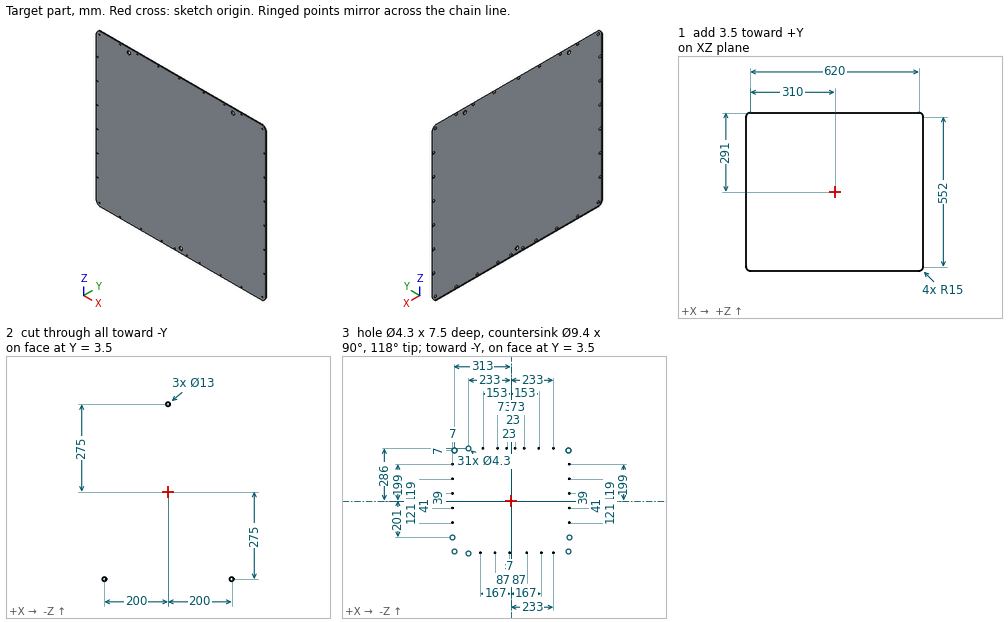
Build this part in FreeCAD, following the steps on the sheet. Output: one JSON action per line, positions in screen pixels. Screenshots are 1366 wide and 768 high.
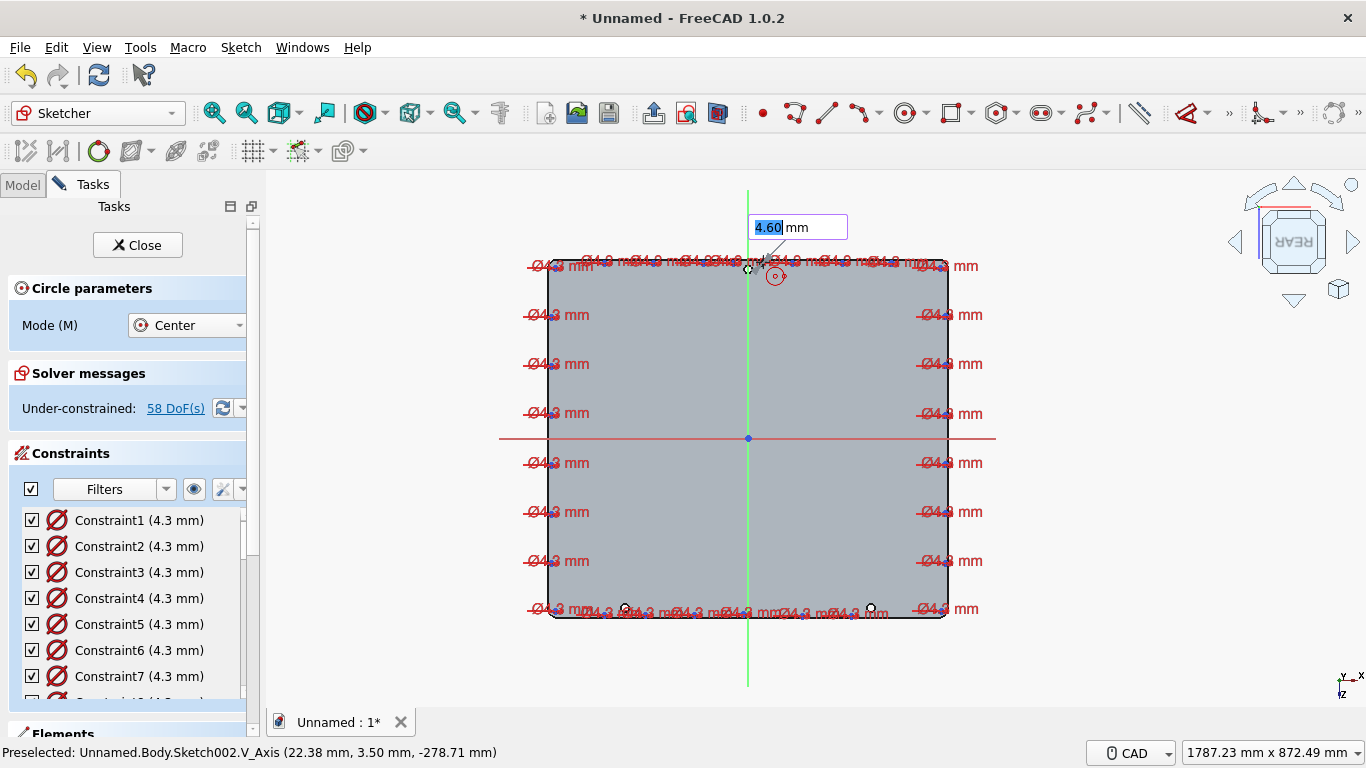
{"action": "type", "text": "4.3"}
{"action": "key", "text": "Return"}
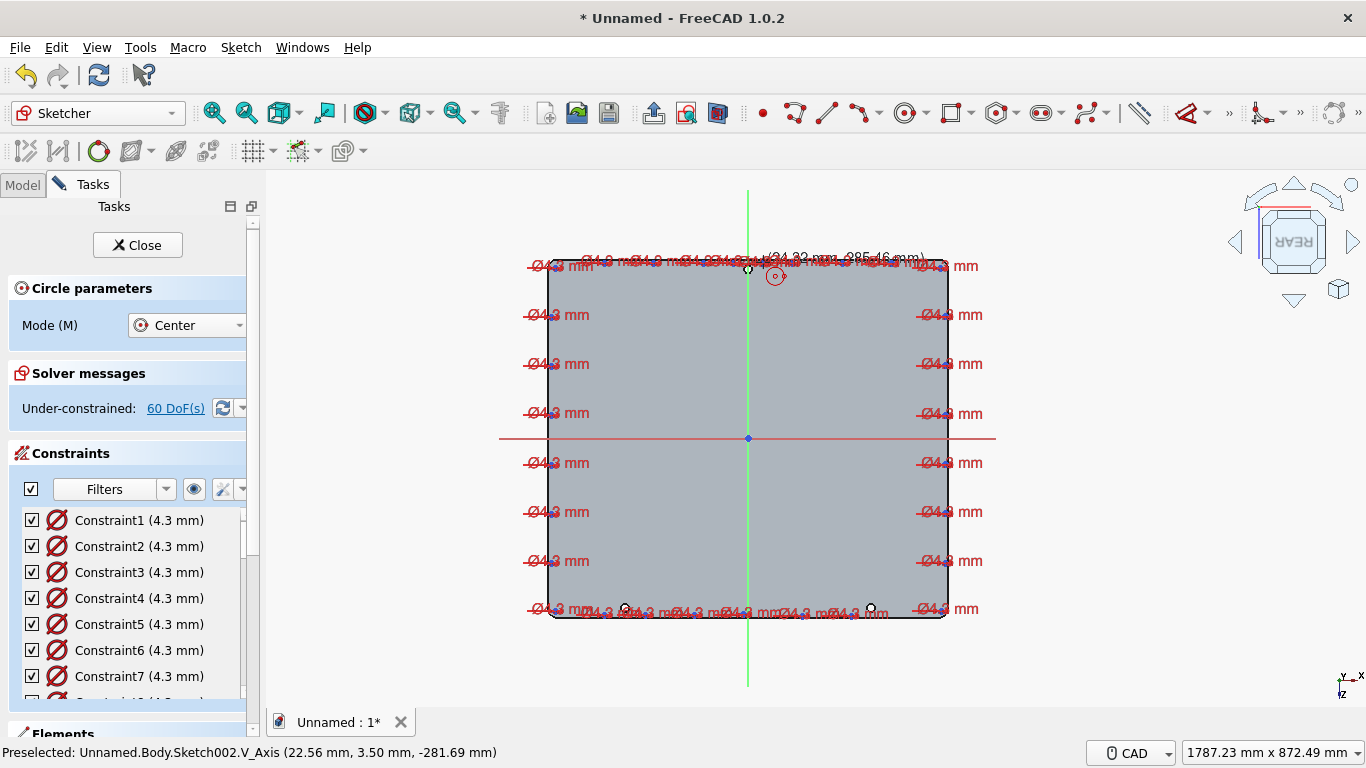
{"action": "scroll", "coordinate": [891, 615], "scroll_direction": "up", "scroll_amount": 15}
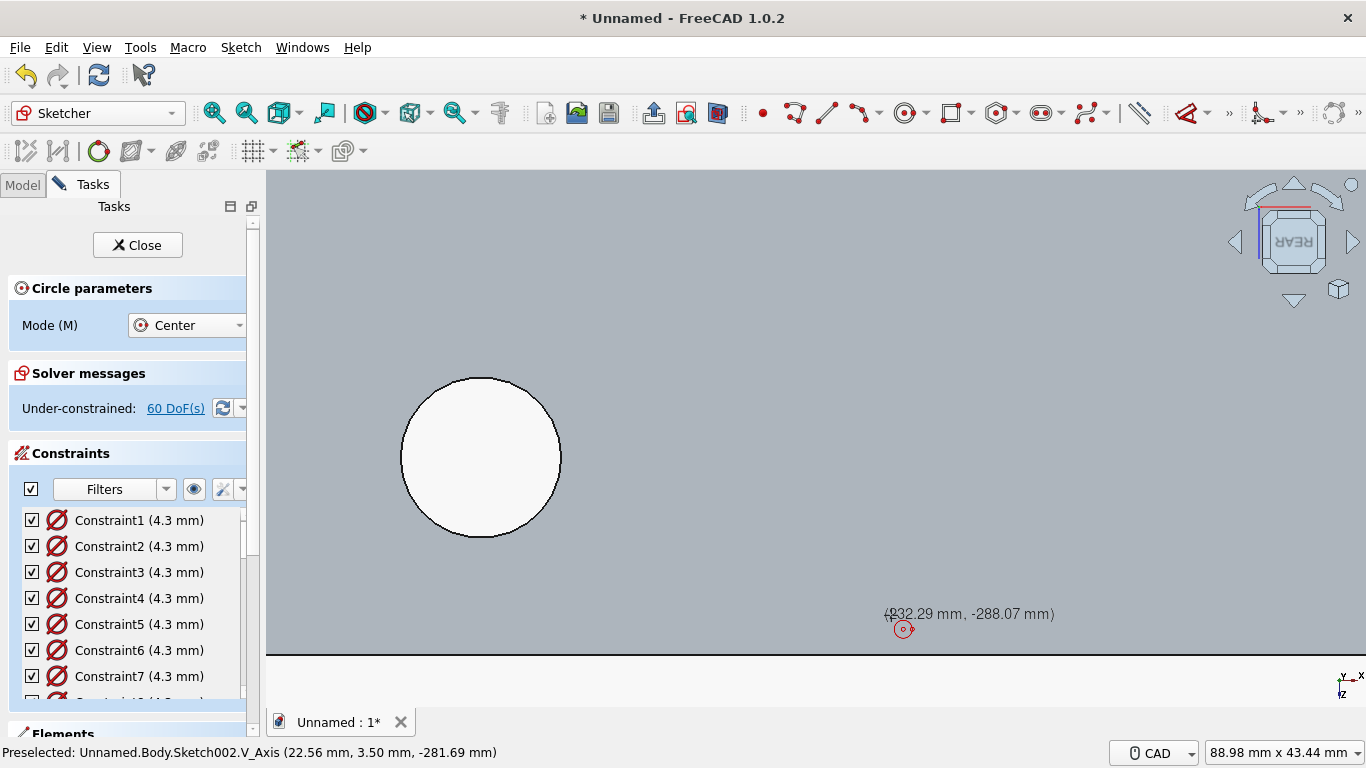
{"action": "scroll", "coordinate": [891, 616], "scroll_direction": "down", "scroll_amount": 15}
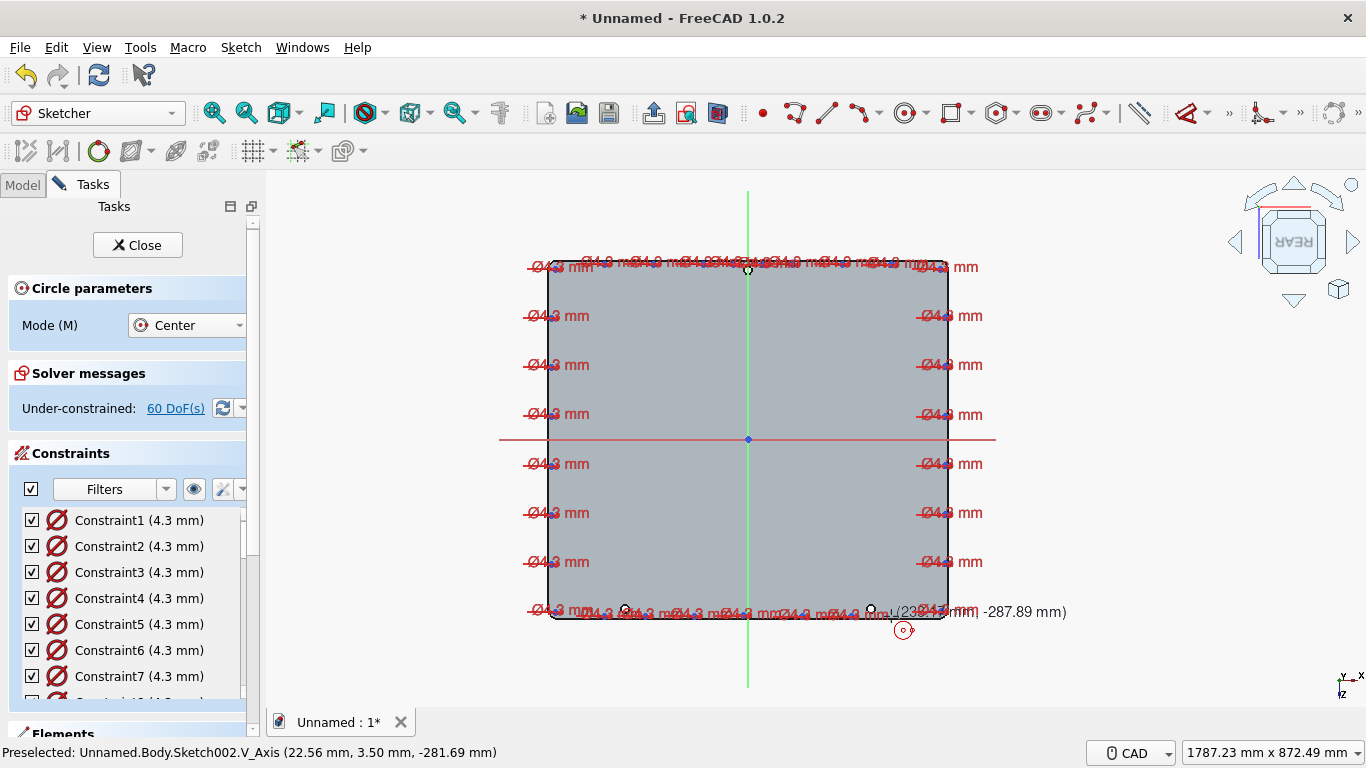
{"action": "left_click", "coordinate": [891, 616]}
{"action": "mouse_move", "coordinate": [892, 615]}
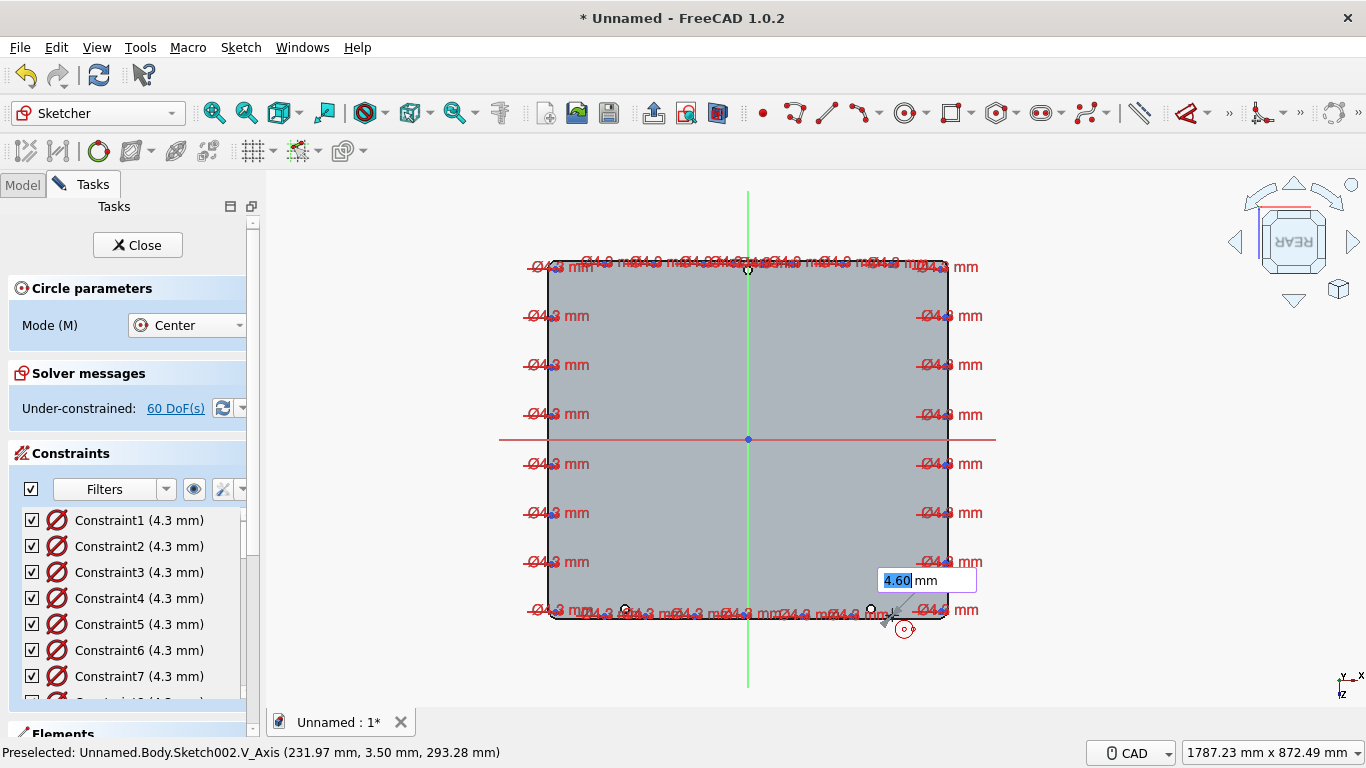
{"action": "type", "text": "4.3"}
{"action": "key", "text": "Return"}
{"action": "key", "text": "Escape"}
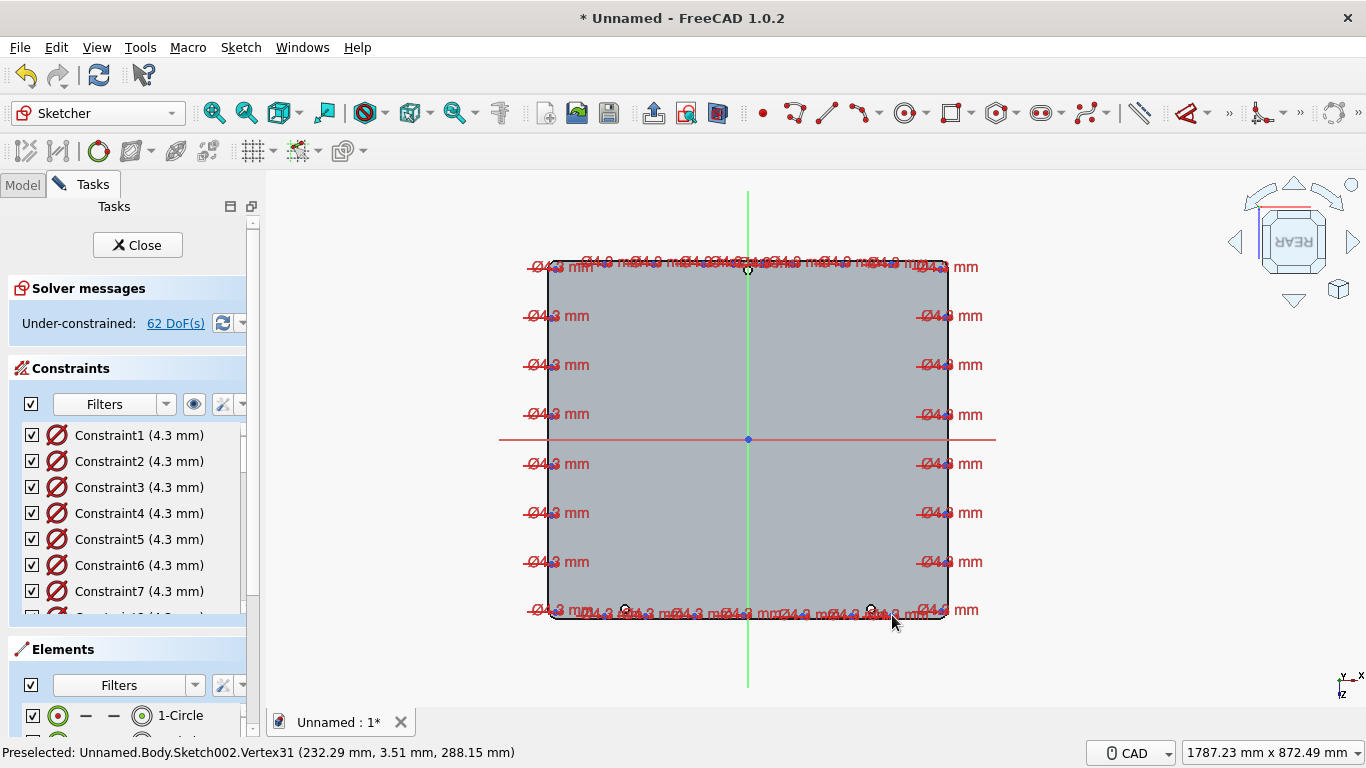
{"action": "left_click", "coordinate": [605, 264]}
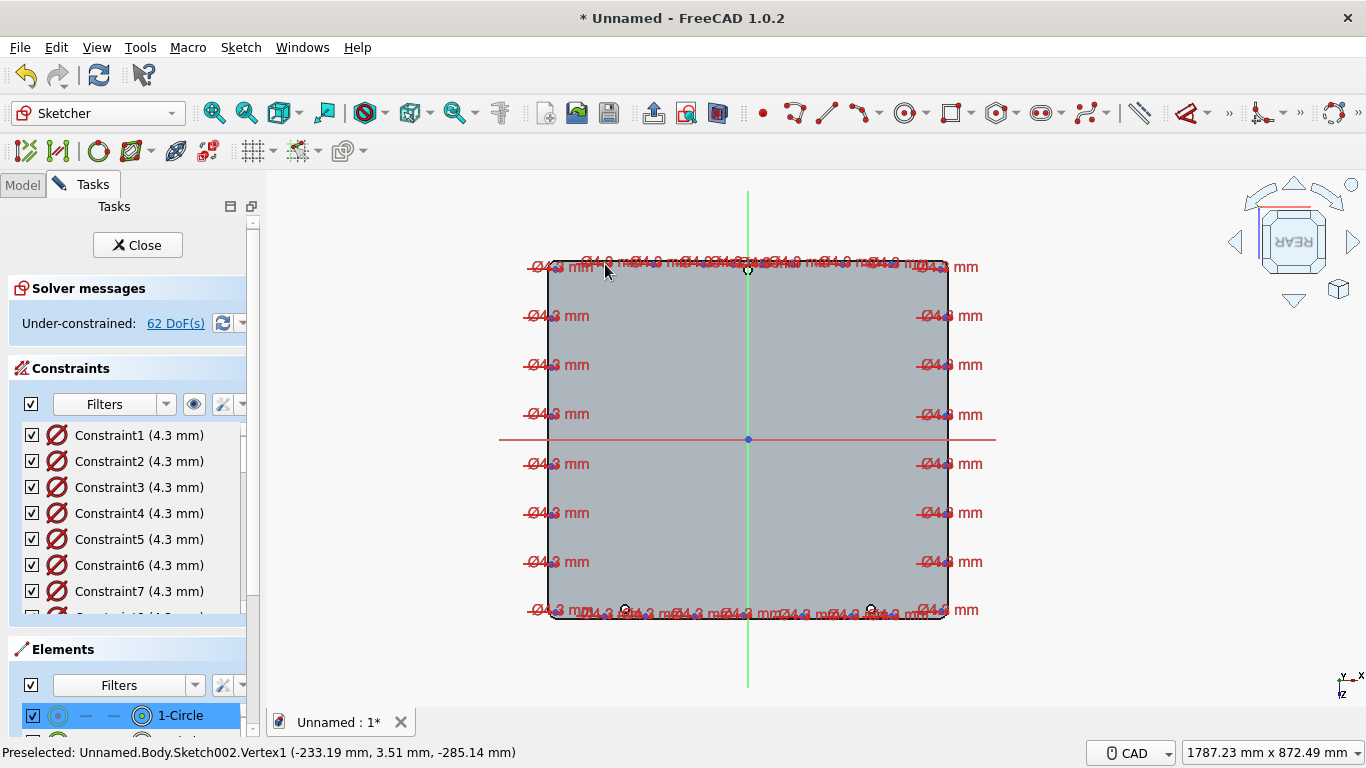
{"action": "left_click", "coordinate": [654, 264]}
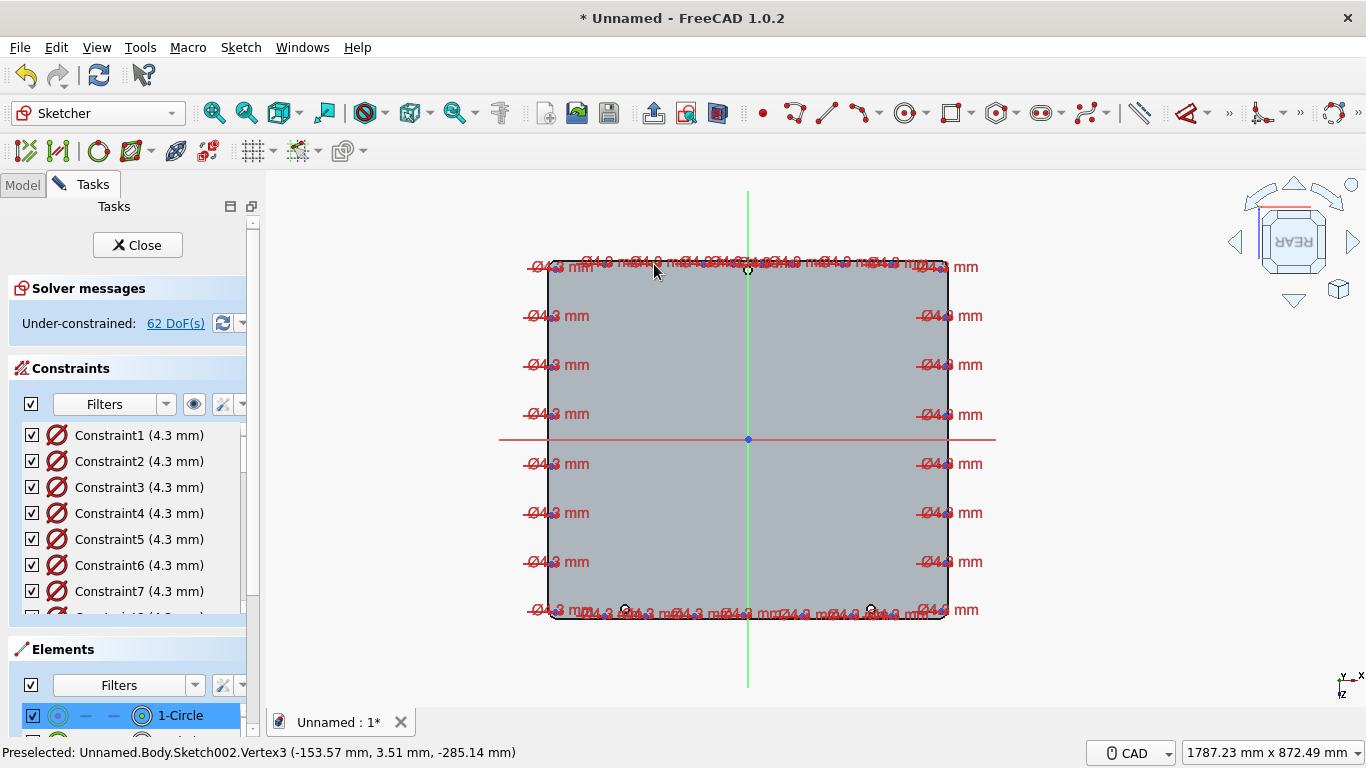
{"action": "key", "text": "h"}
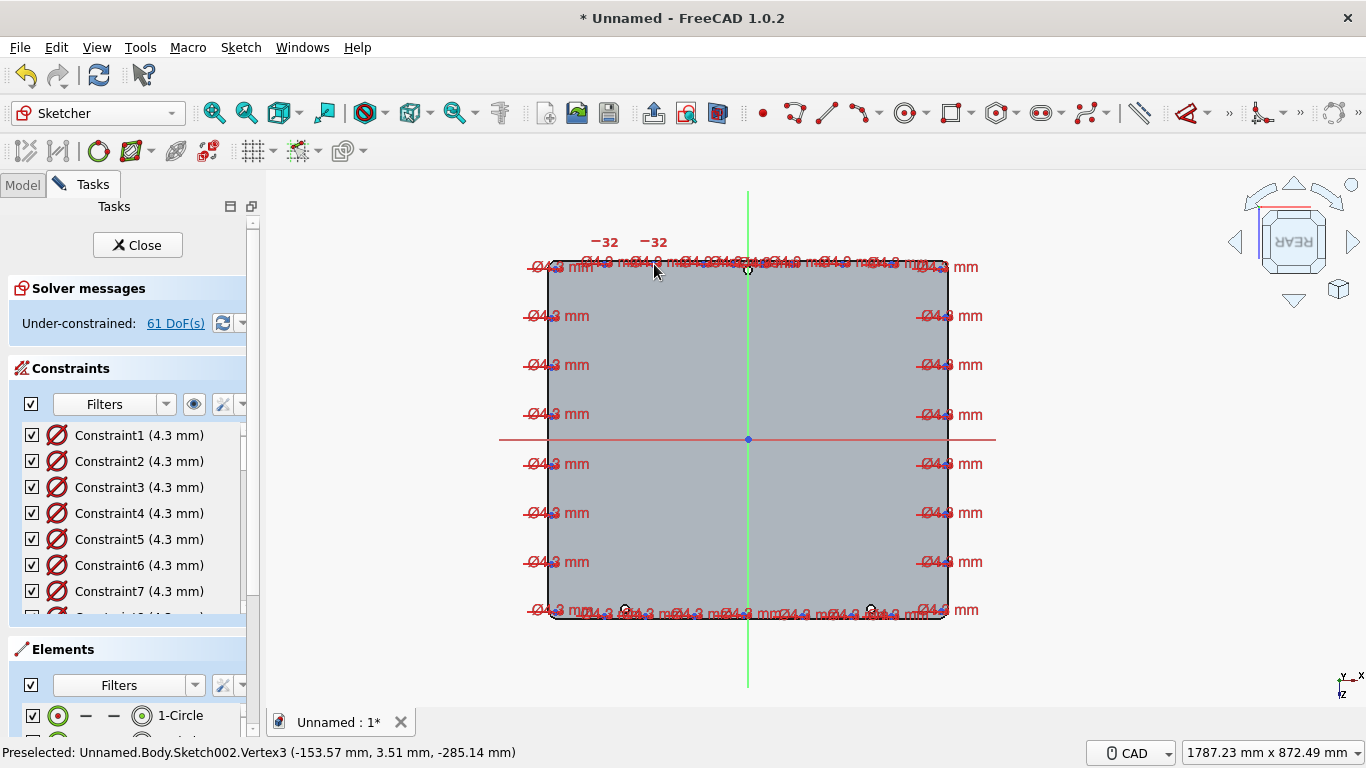
{"action": "left_click", "coordinate": [654, 264]}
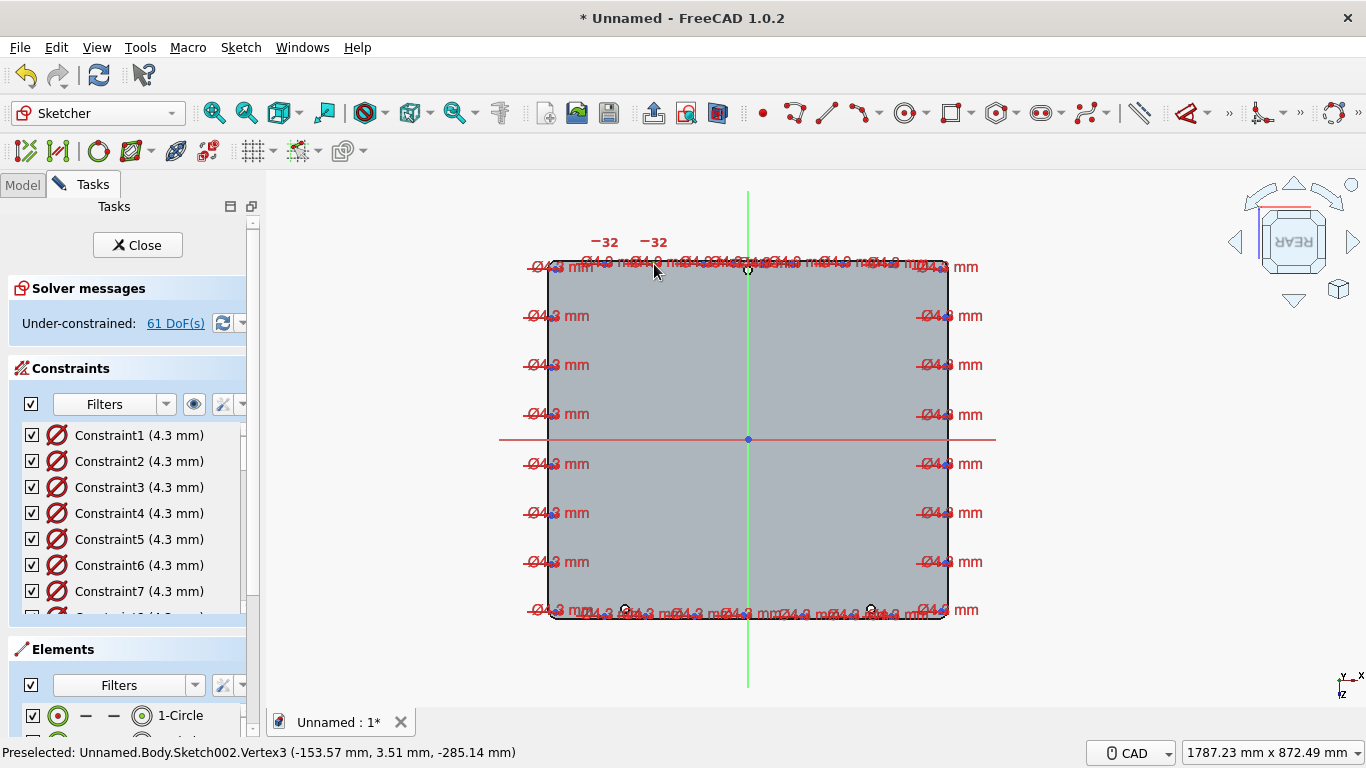
{"action": "left_click", "coordinate": [704, 264]}